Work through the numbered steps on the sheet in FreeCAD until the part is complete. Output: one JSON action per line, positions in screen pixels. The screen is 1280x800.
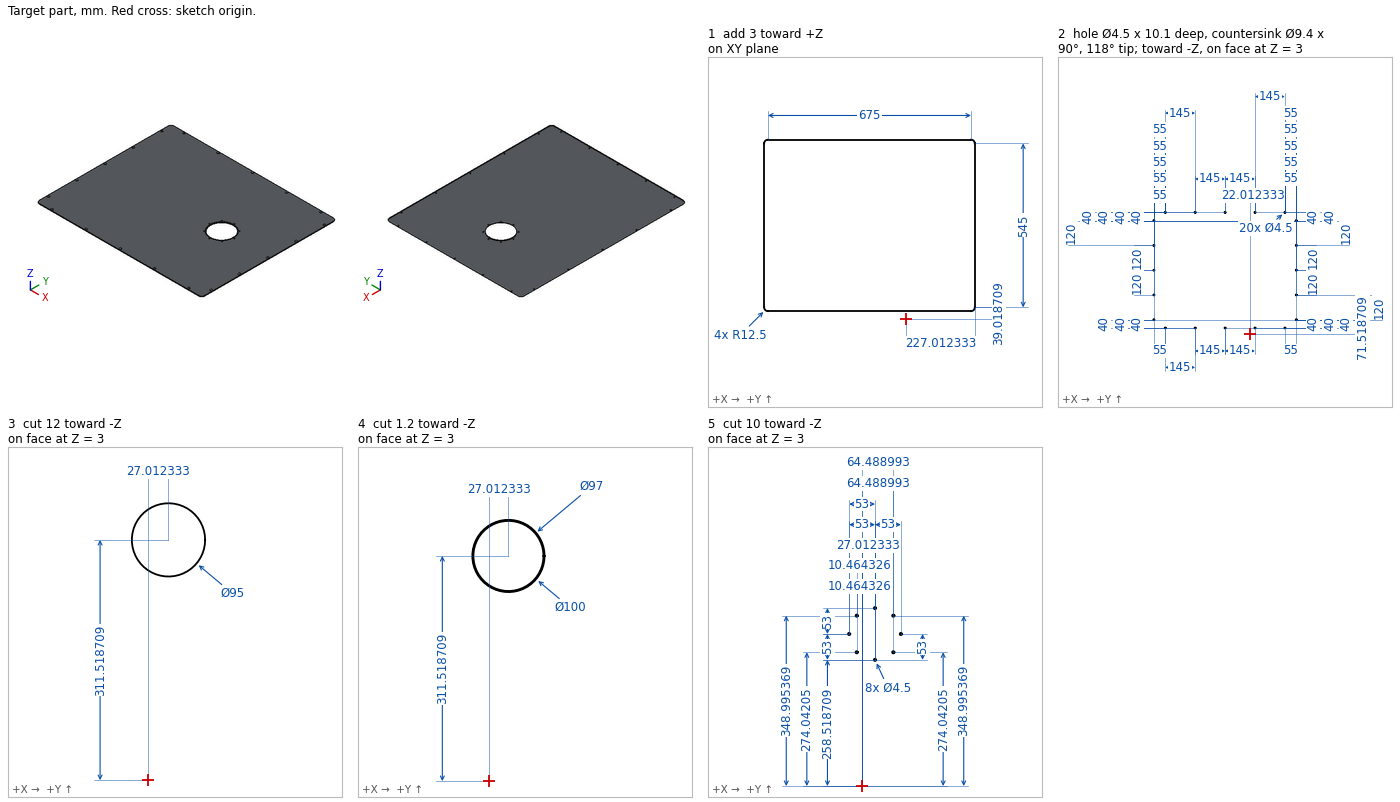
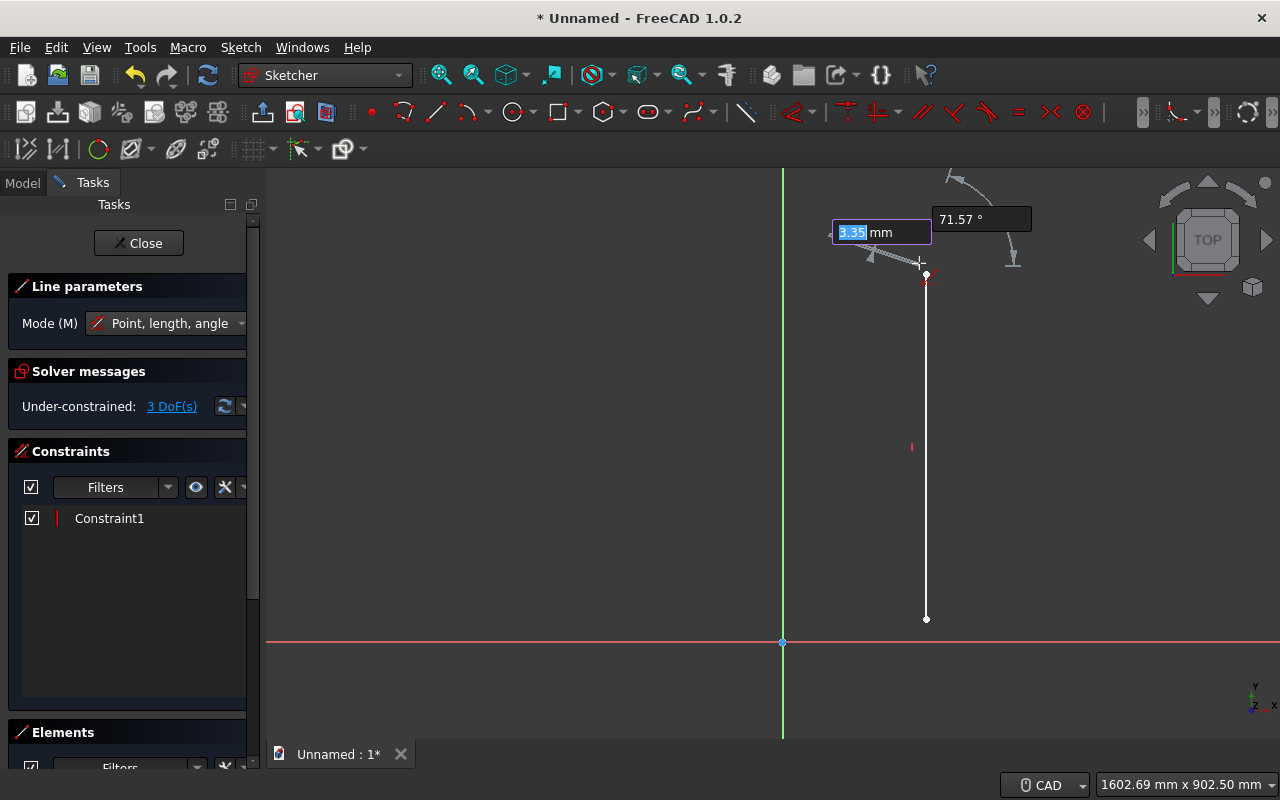
{"action": "left_click", "coordinate": [491, 265]}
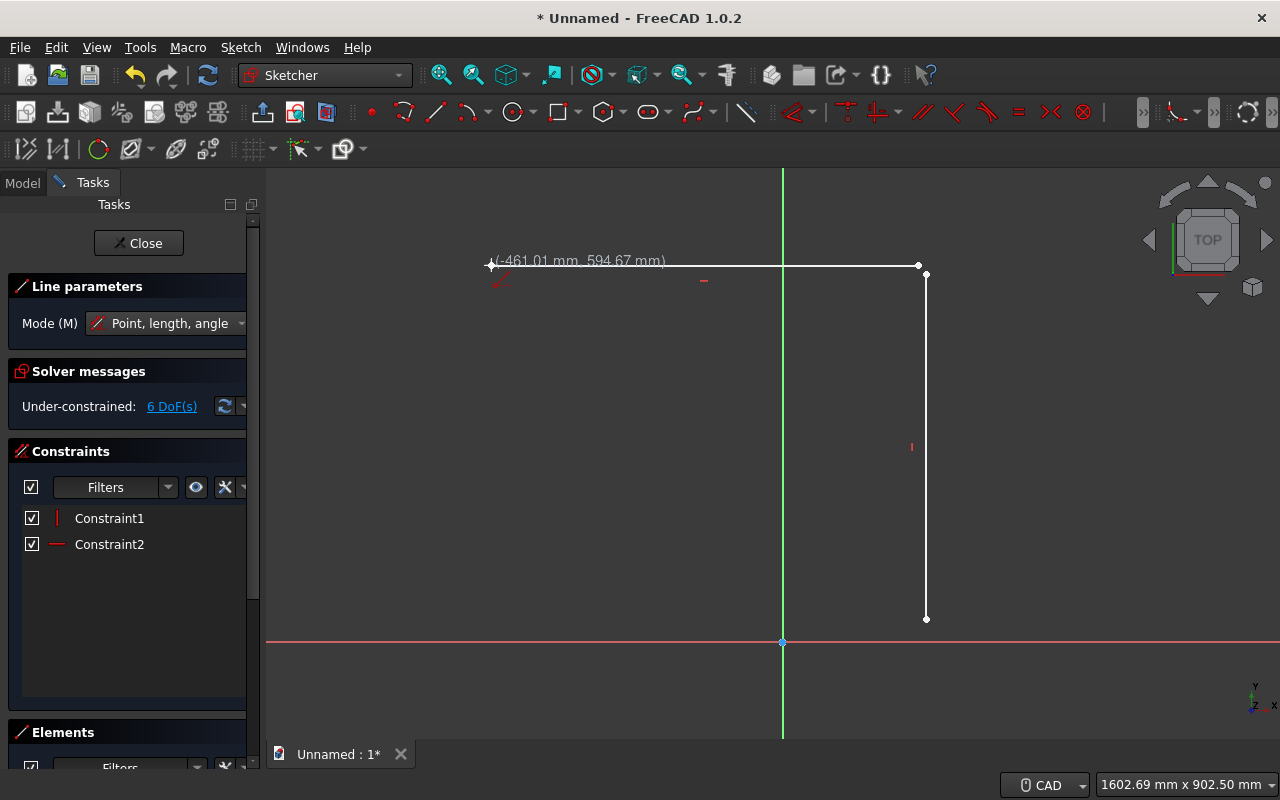
{"action": "scroll", "coordinate": [483, 273], "scroll_direction": "up", "scroll_amount": 2}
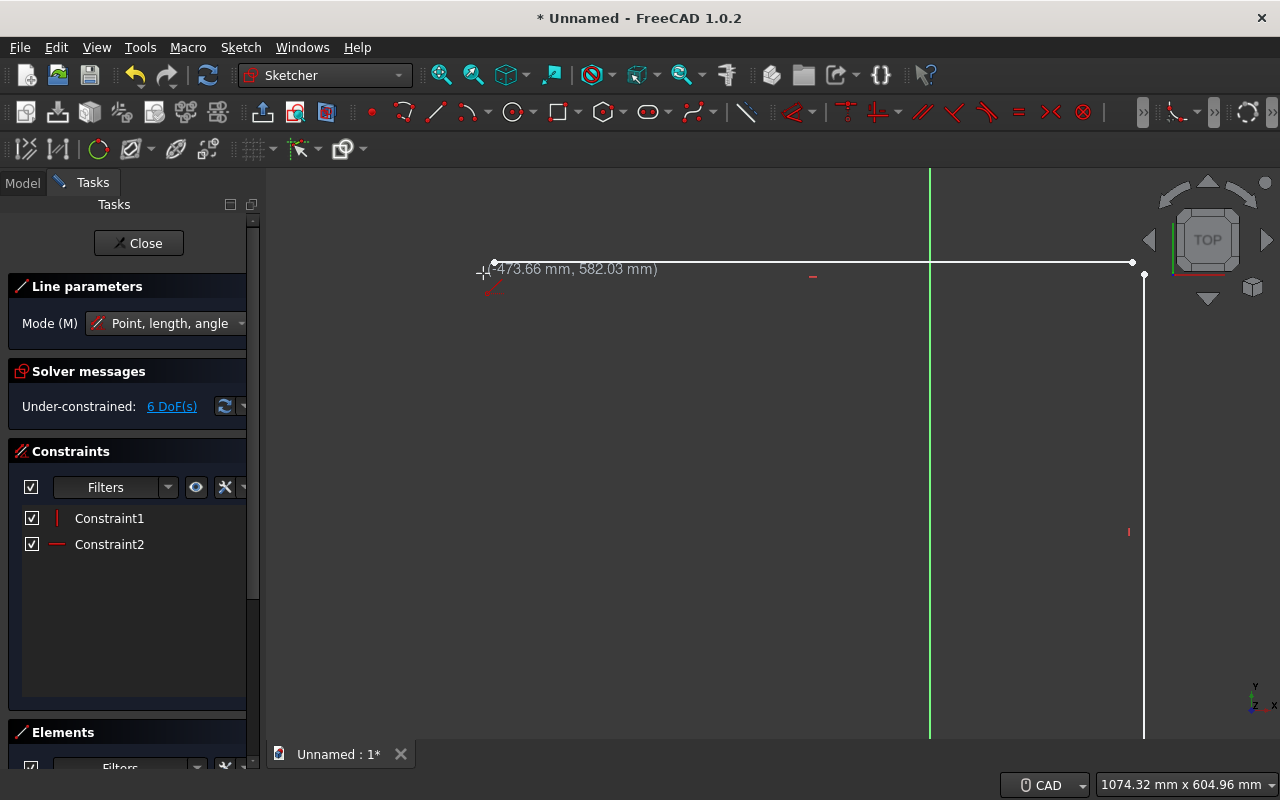
{"action": "left_click", "coordinate": [484, 273]}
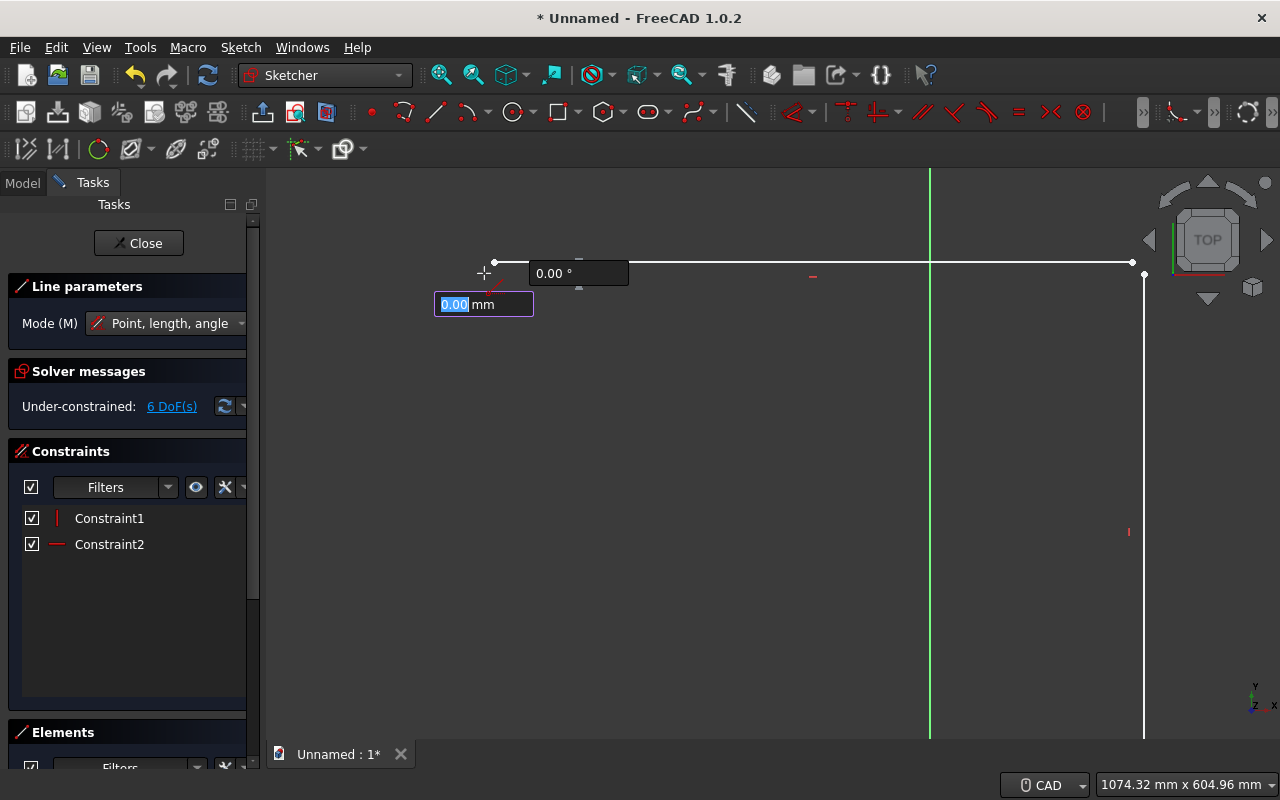
{"action": "scroll", "coordinate": [482, 273], "scroll_direction": "down", "scroll_amount": 2}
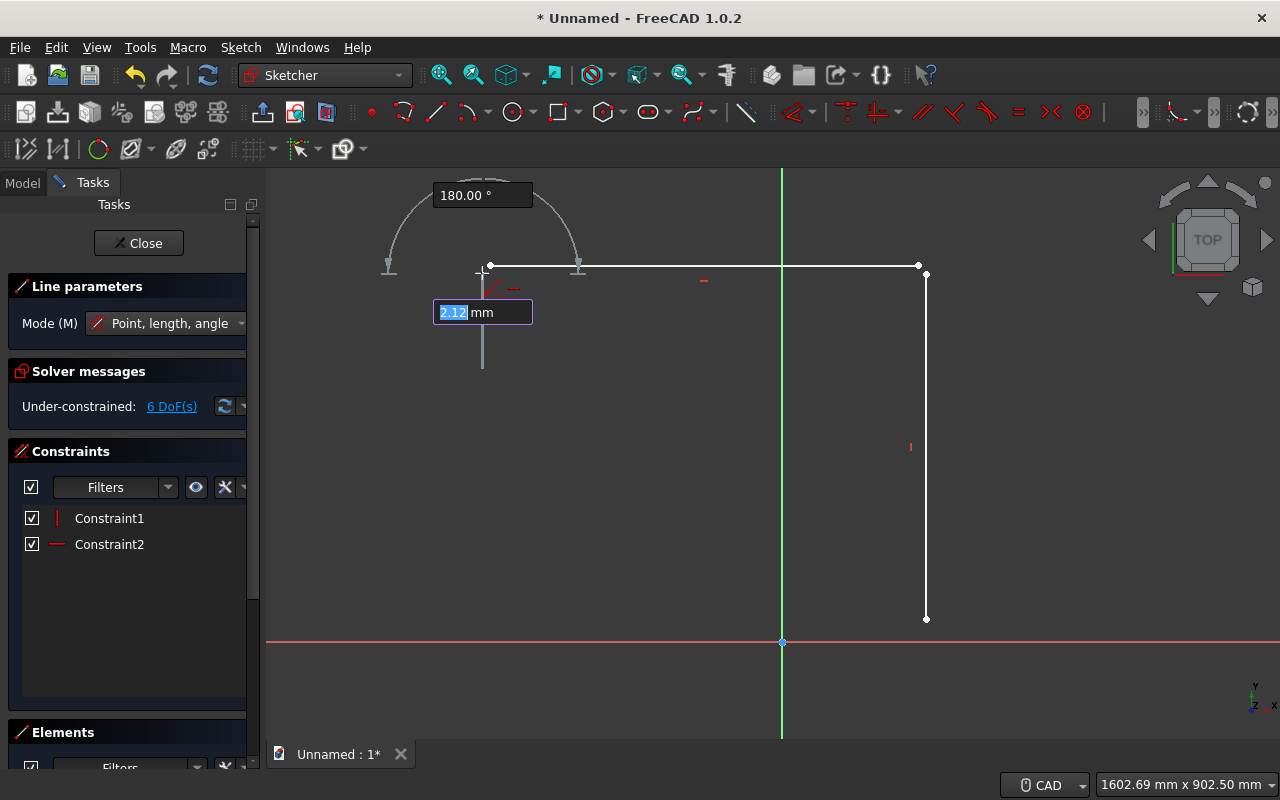
{"action": "left_click", "coordinate": [483, 618]}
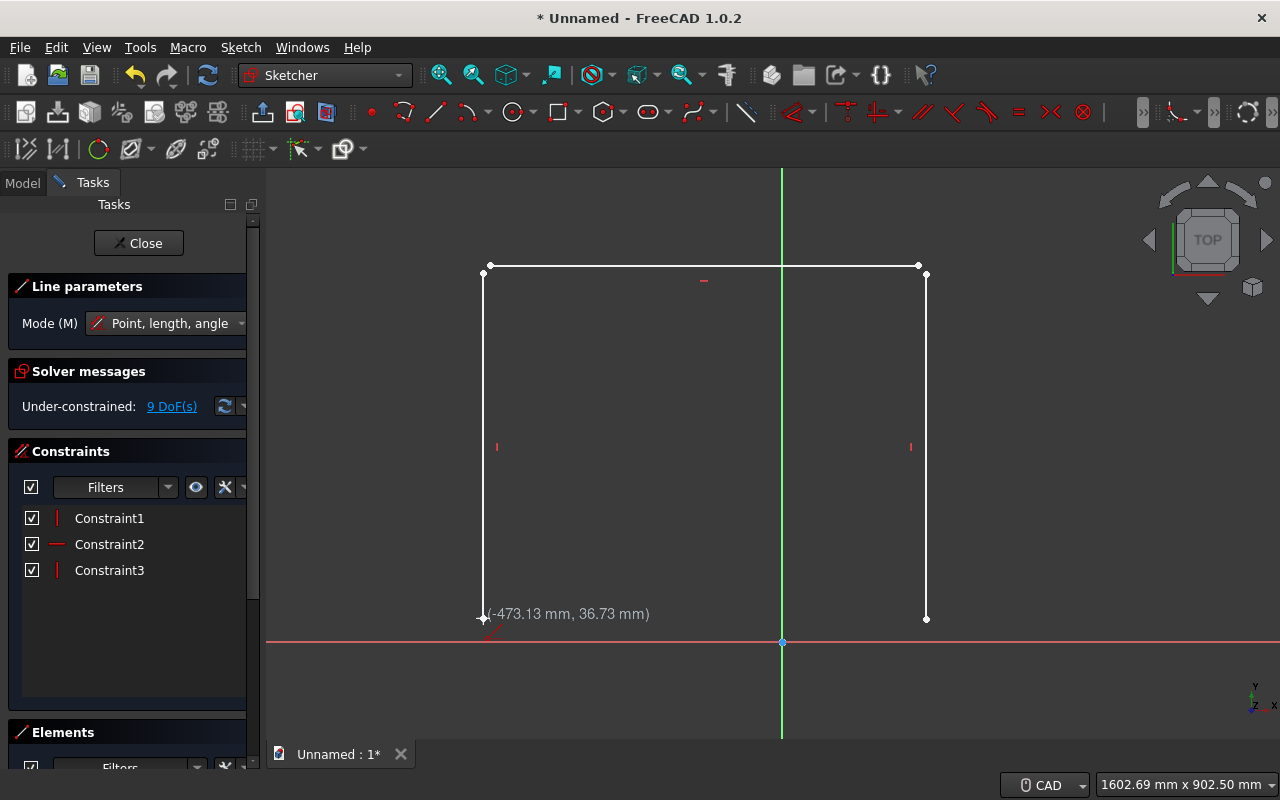
{"action": "scroll", "coordinate": [491, 625], "scroll_direction": "up", "scroll_amount": 2}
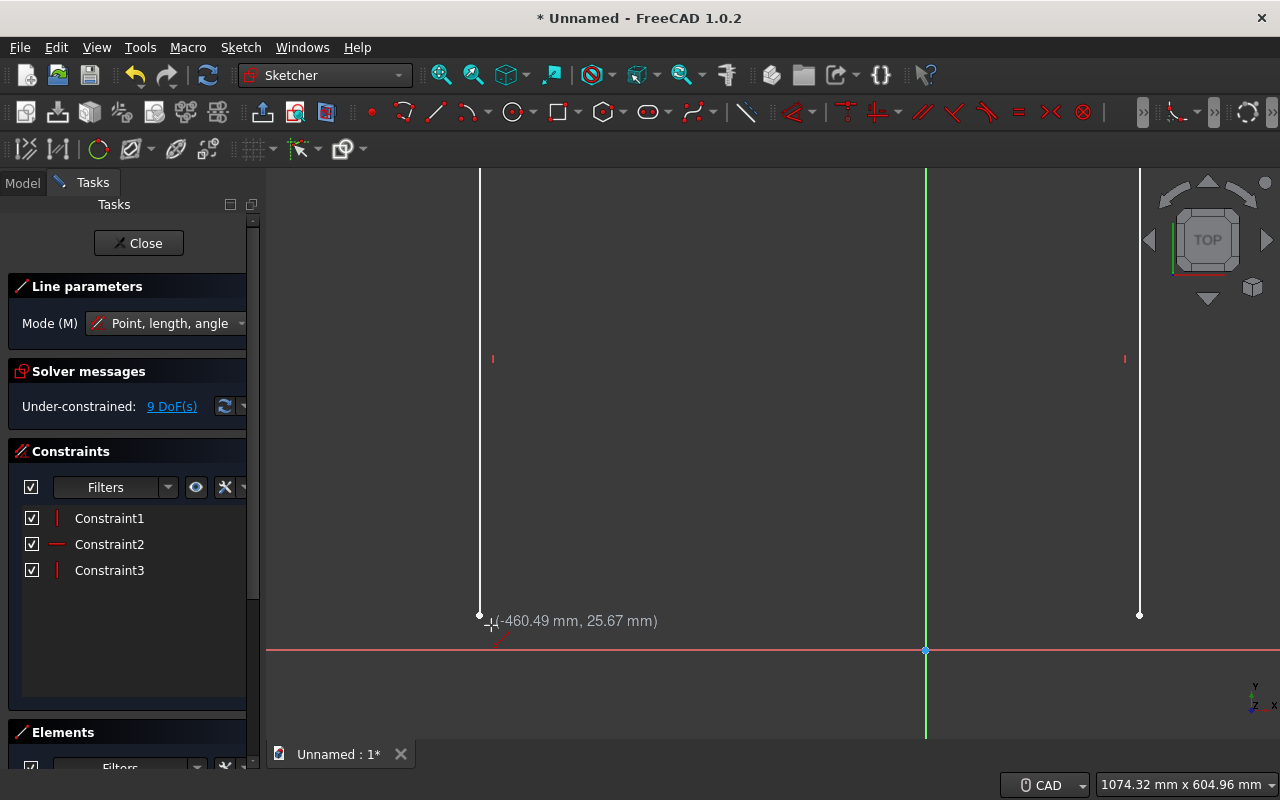
{"action": "left_click", "coordinate": [491, 625]}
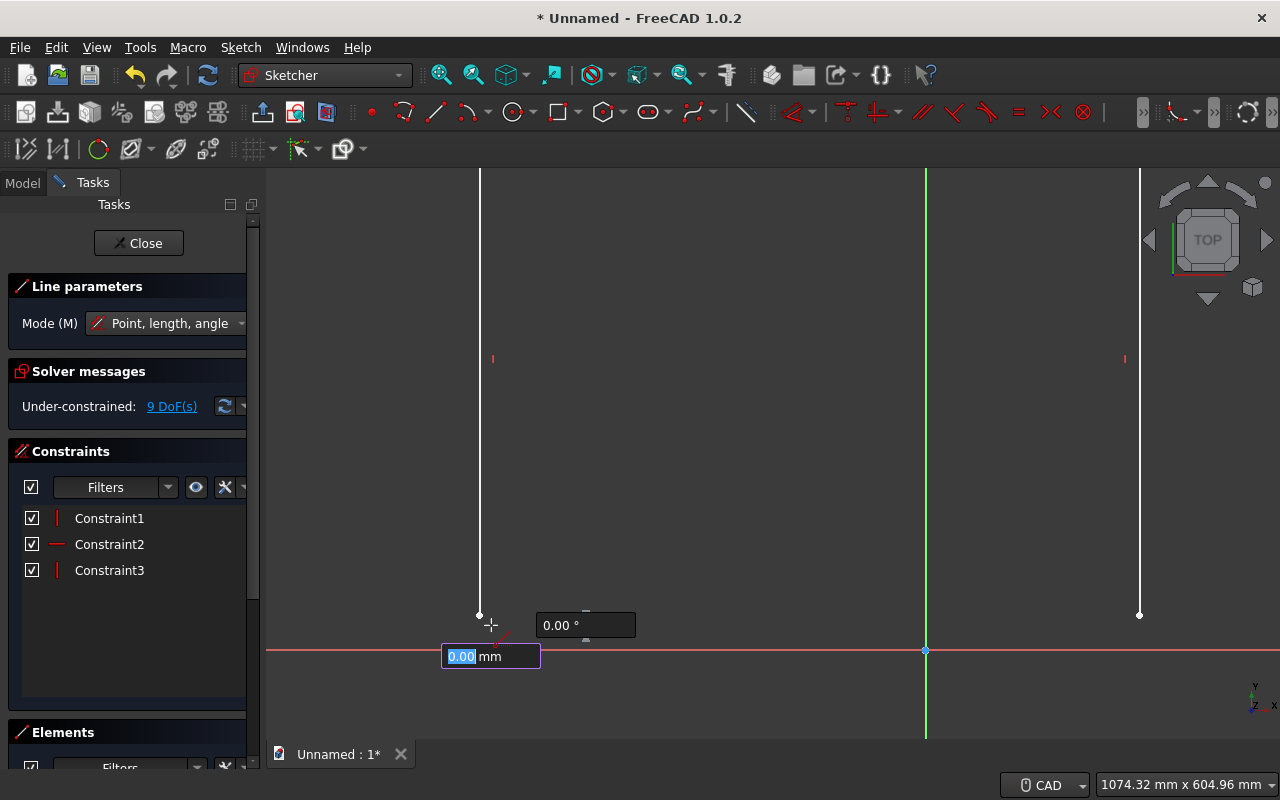
{"action": "scroll", "coordinate": [491, 626], "scroll_direction": "down", "scroll_amount": 2}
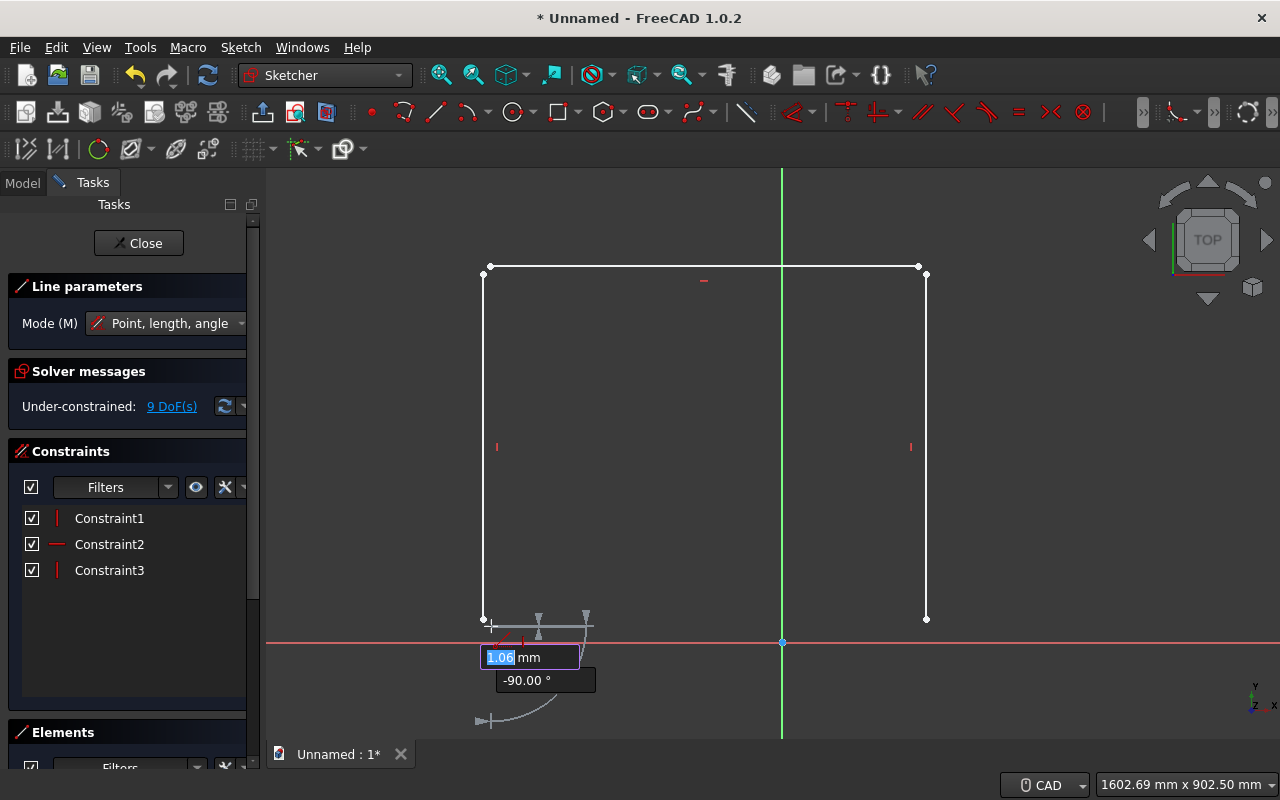
{"action": "scroll", "coordinate": [918, 626], "scroll_direction": "up", "scroll_amount": 2}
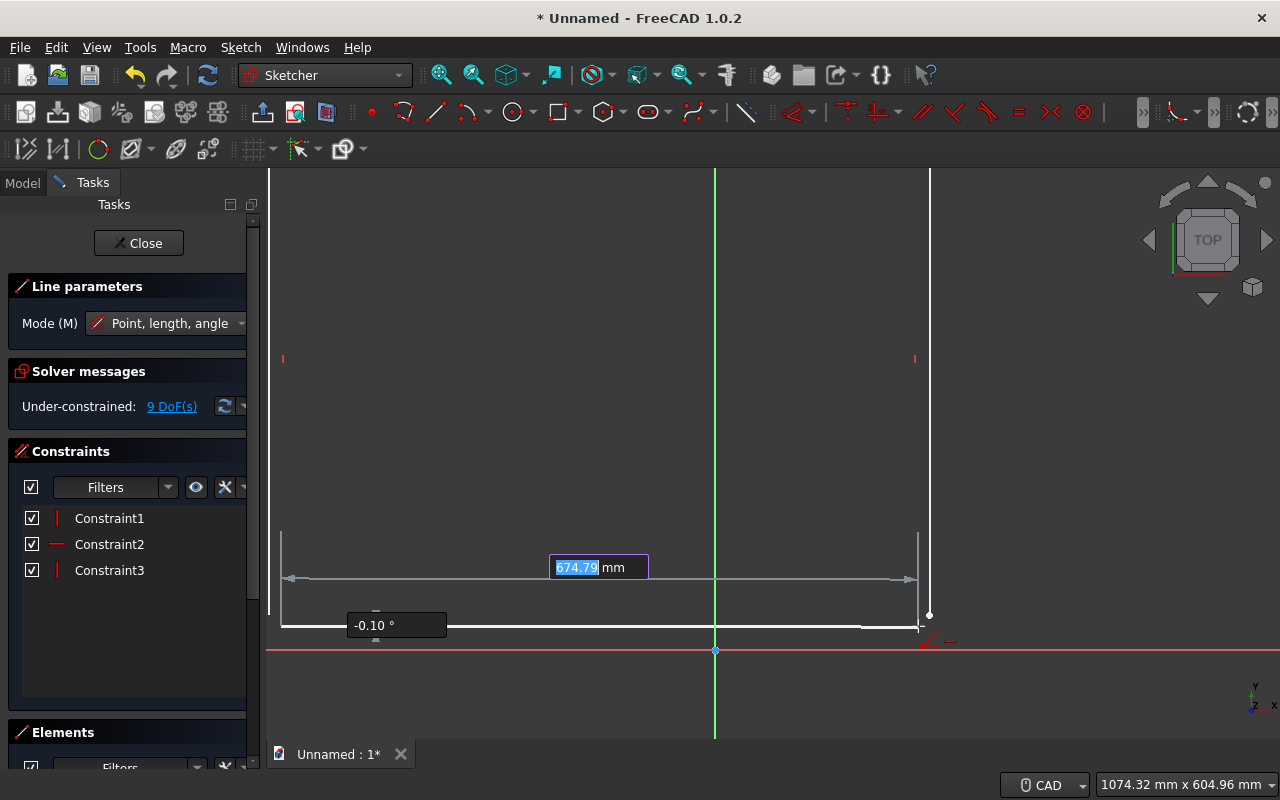
{"action": "left_click", "coordinate": [918, 625]}